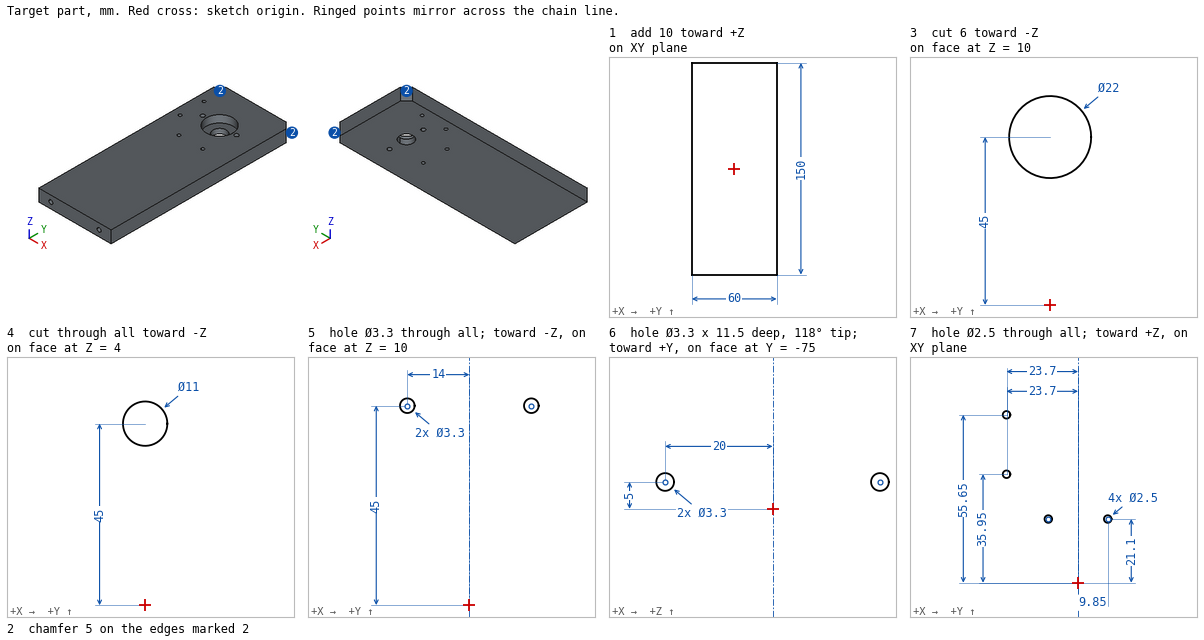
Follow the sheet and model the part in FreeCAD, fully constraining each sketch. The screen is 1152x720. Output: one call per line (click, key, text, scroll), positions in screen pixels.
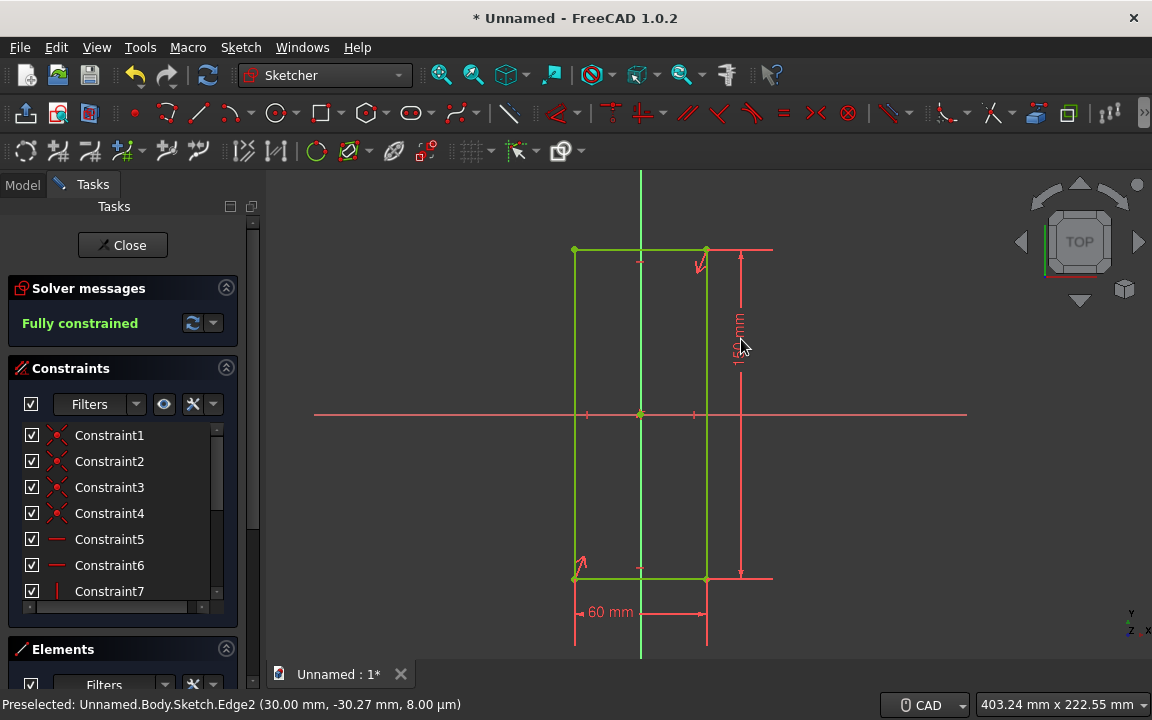
click(123, 245)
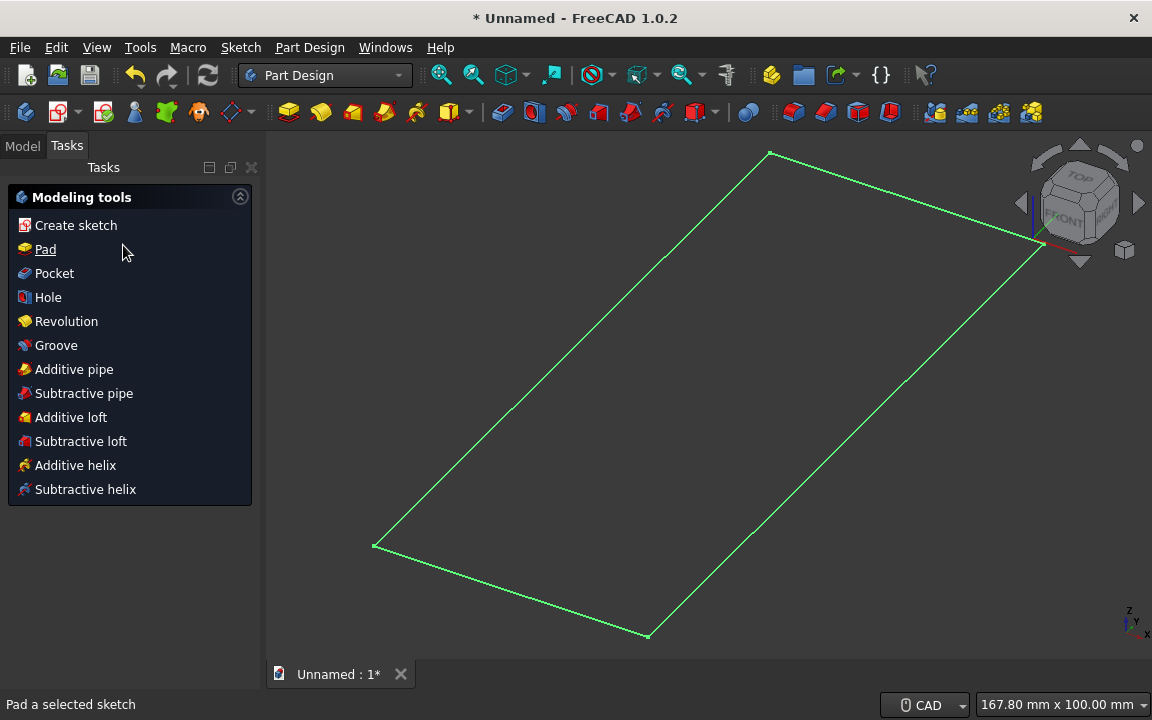
click(290, 112)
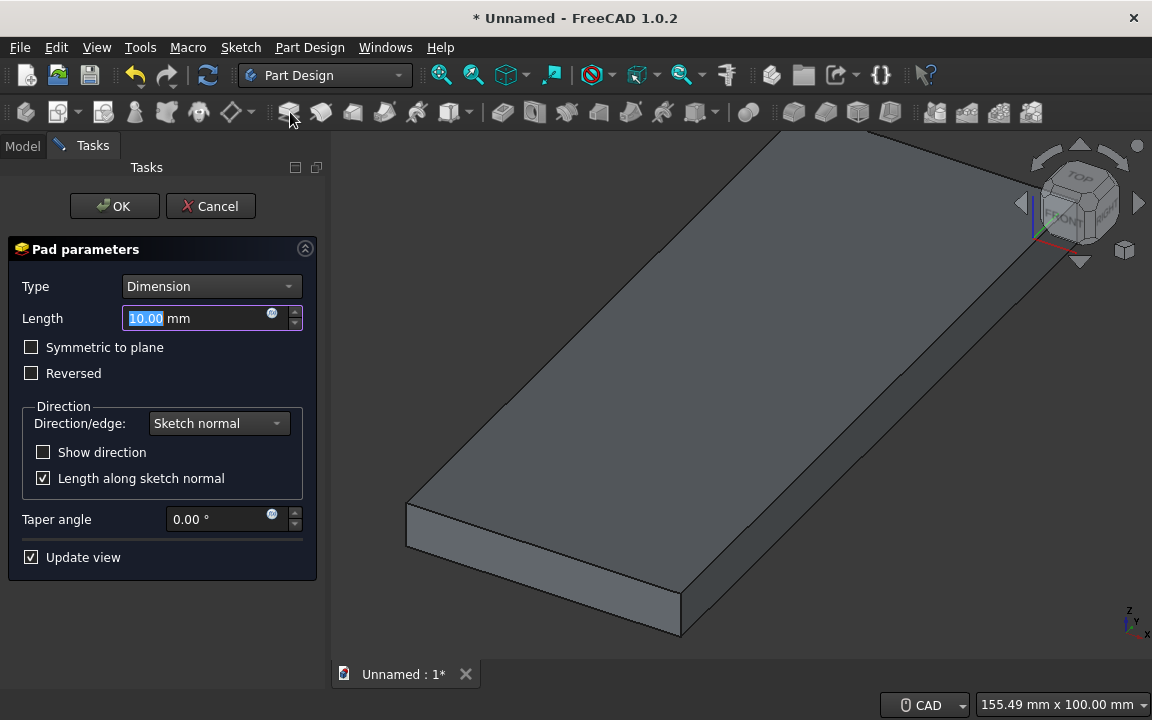
text(10)
key(Tab)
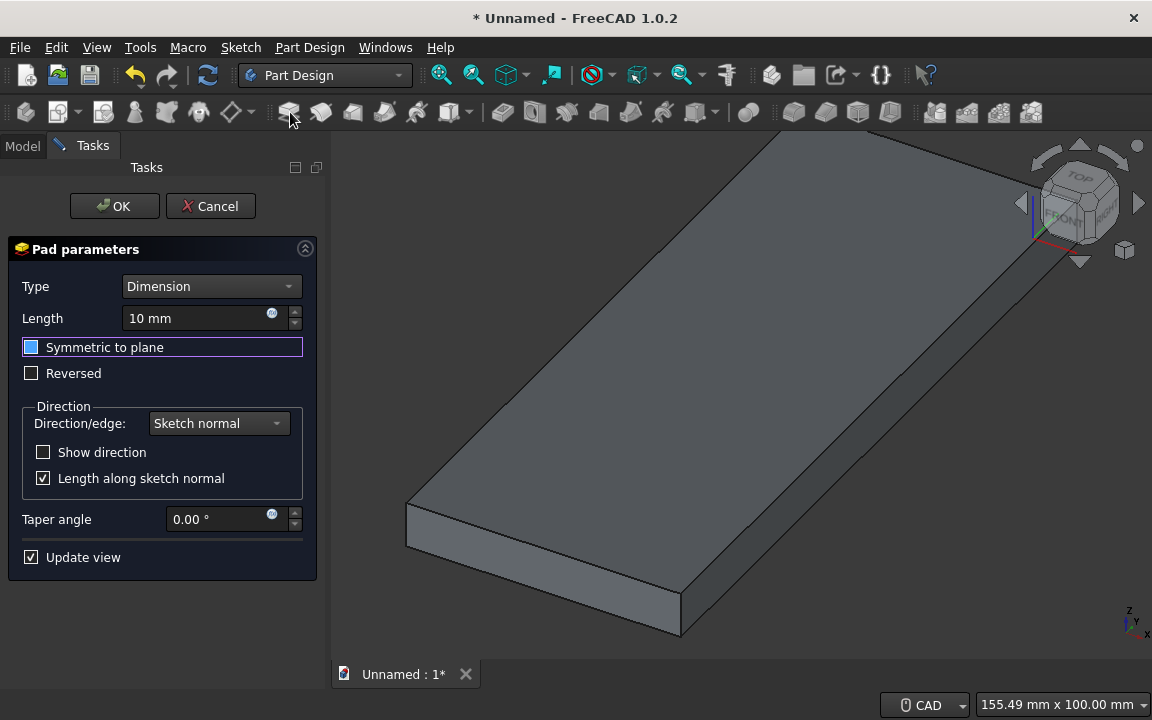
click(115, 206)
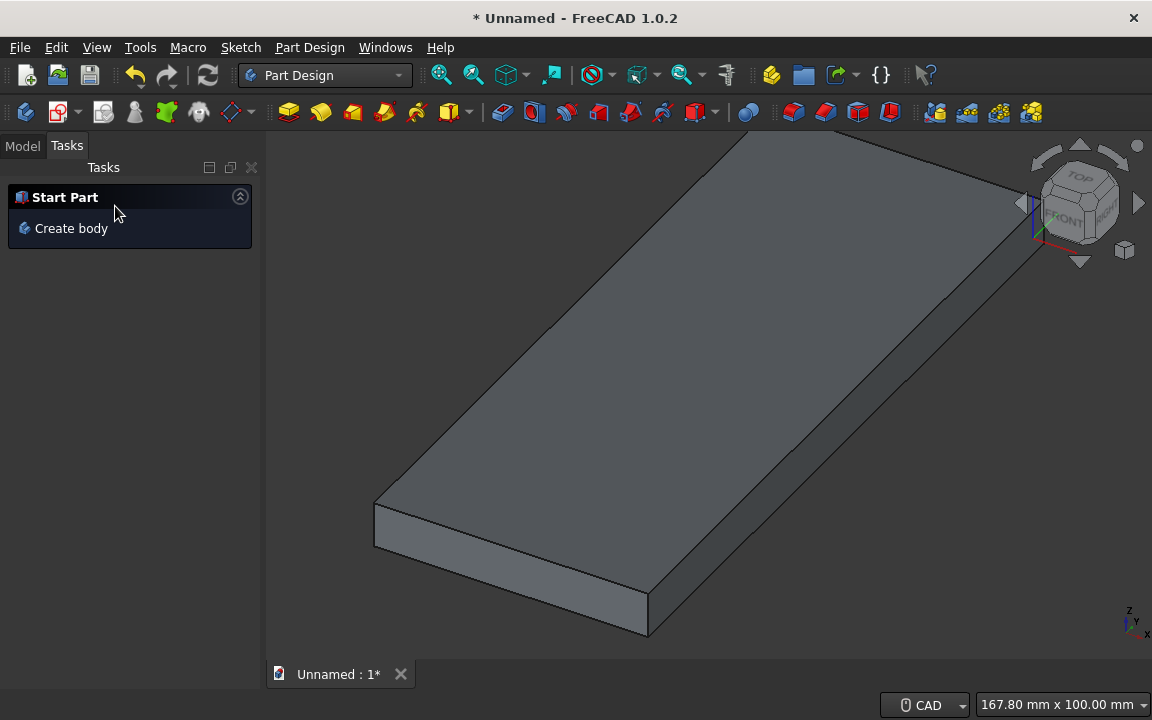
click(442, 76)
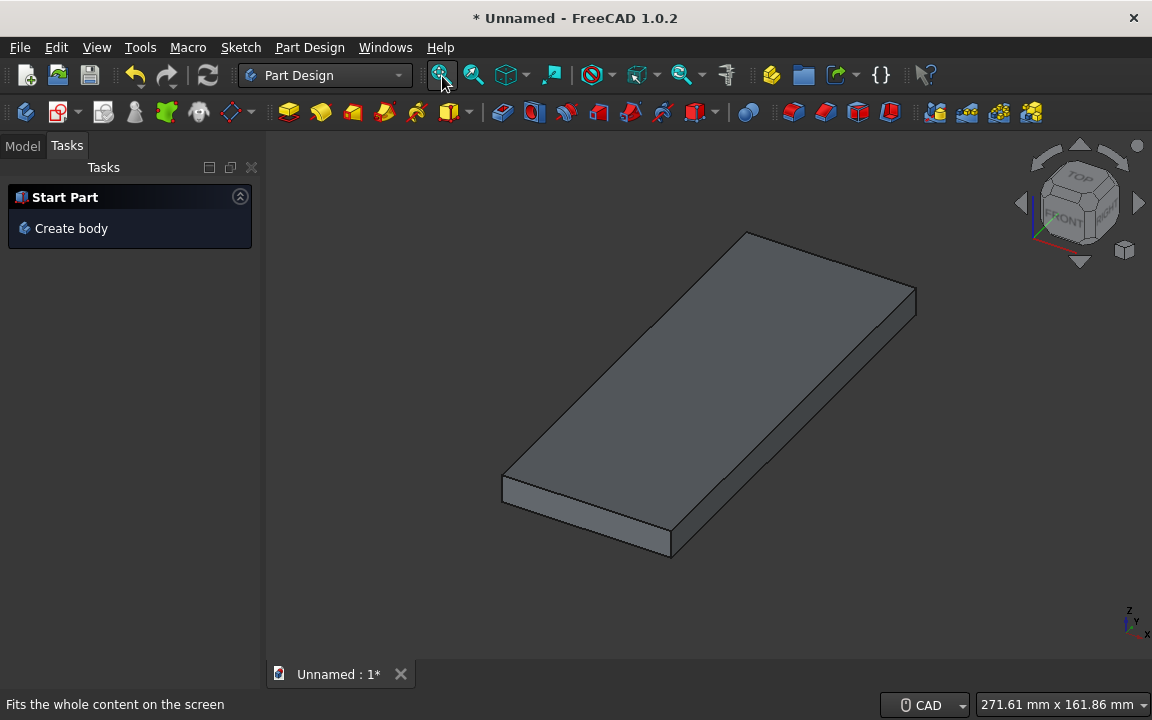
key(0)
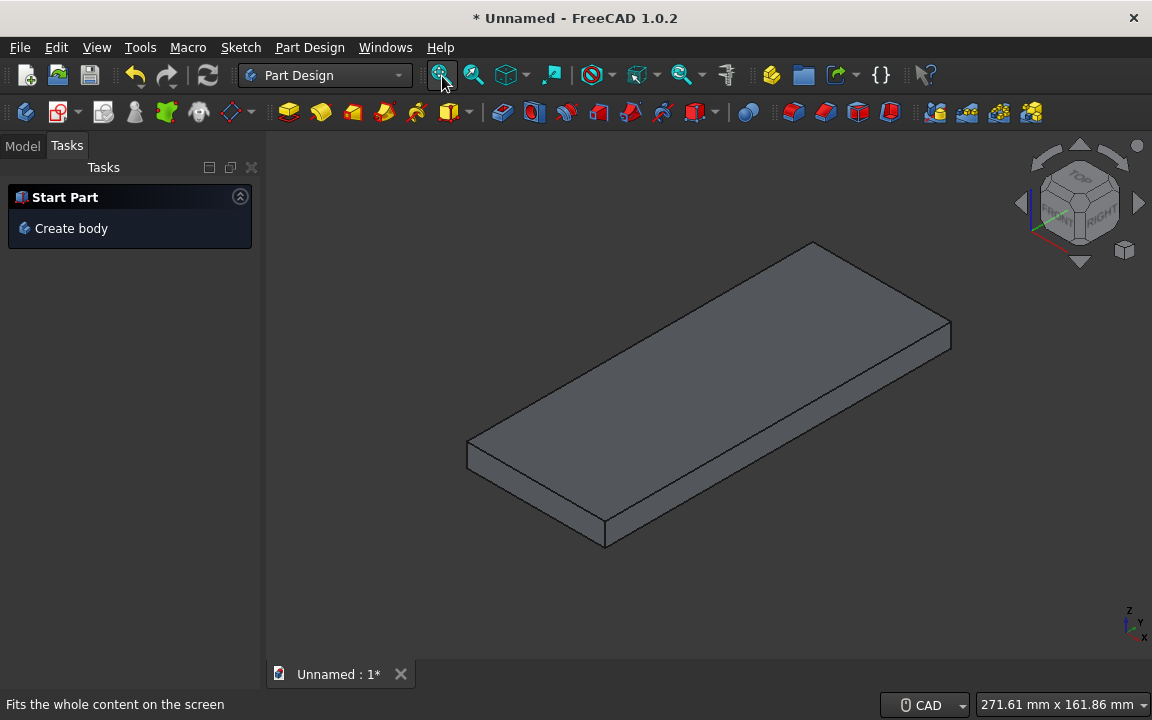
key(2)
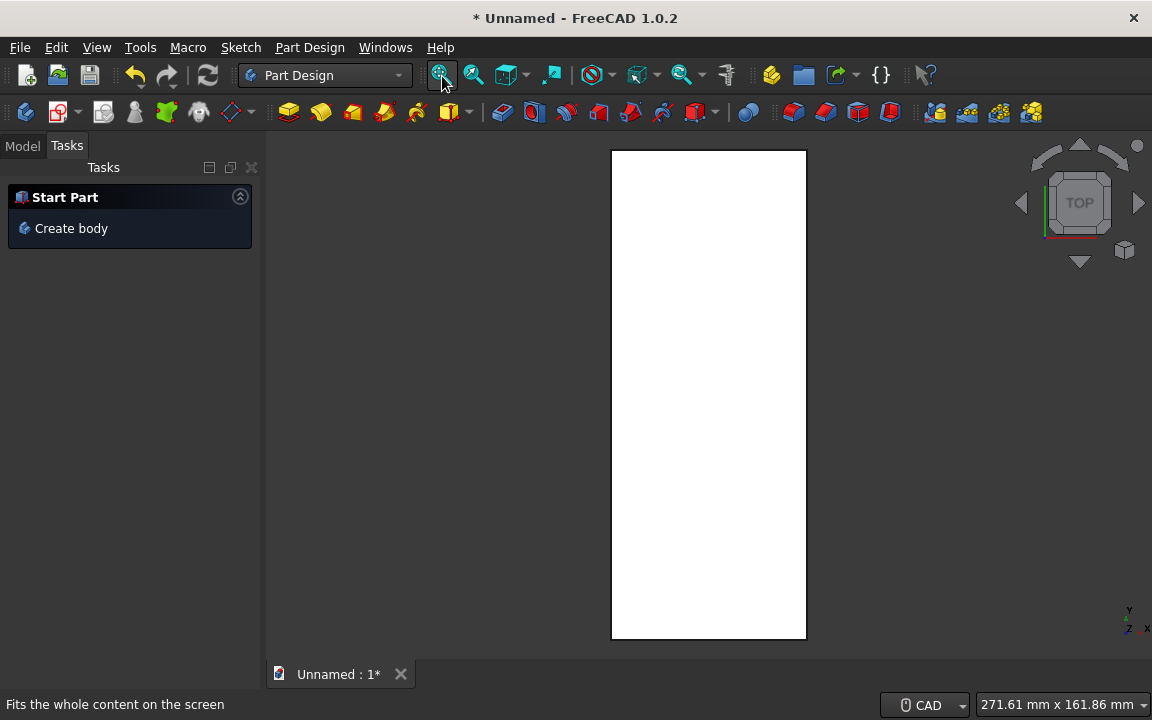
key(1)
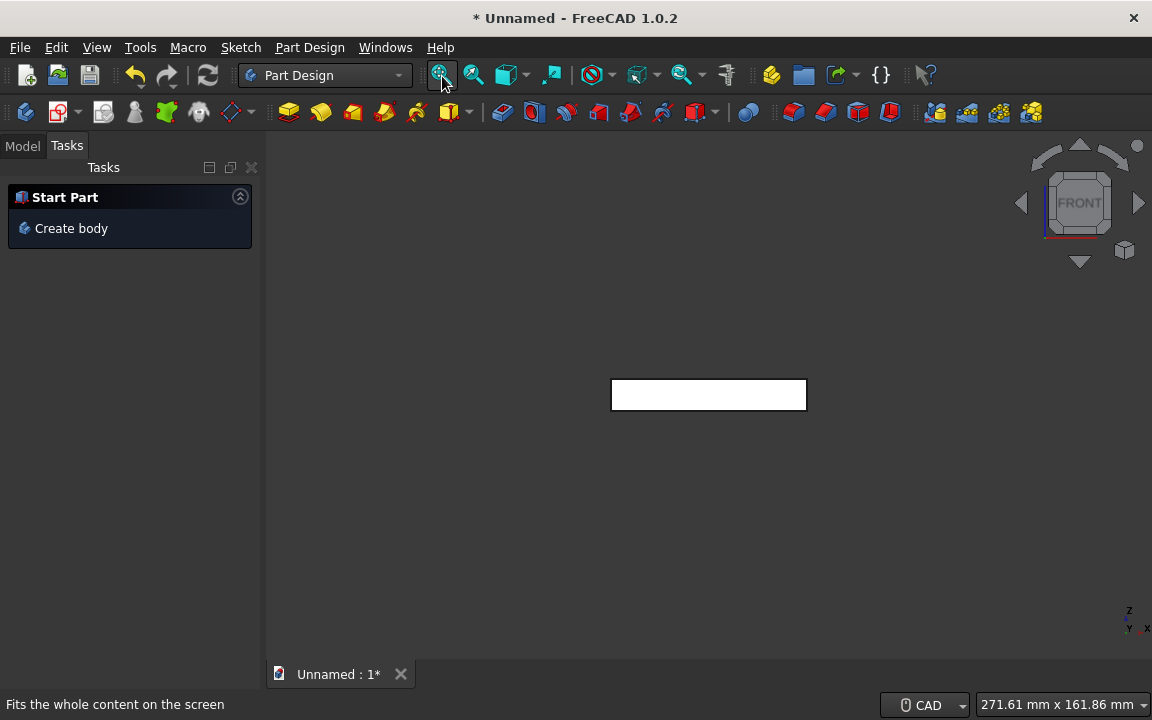
click(442, 76)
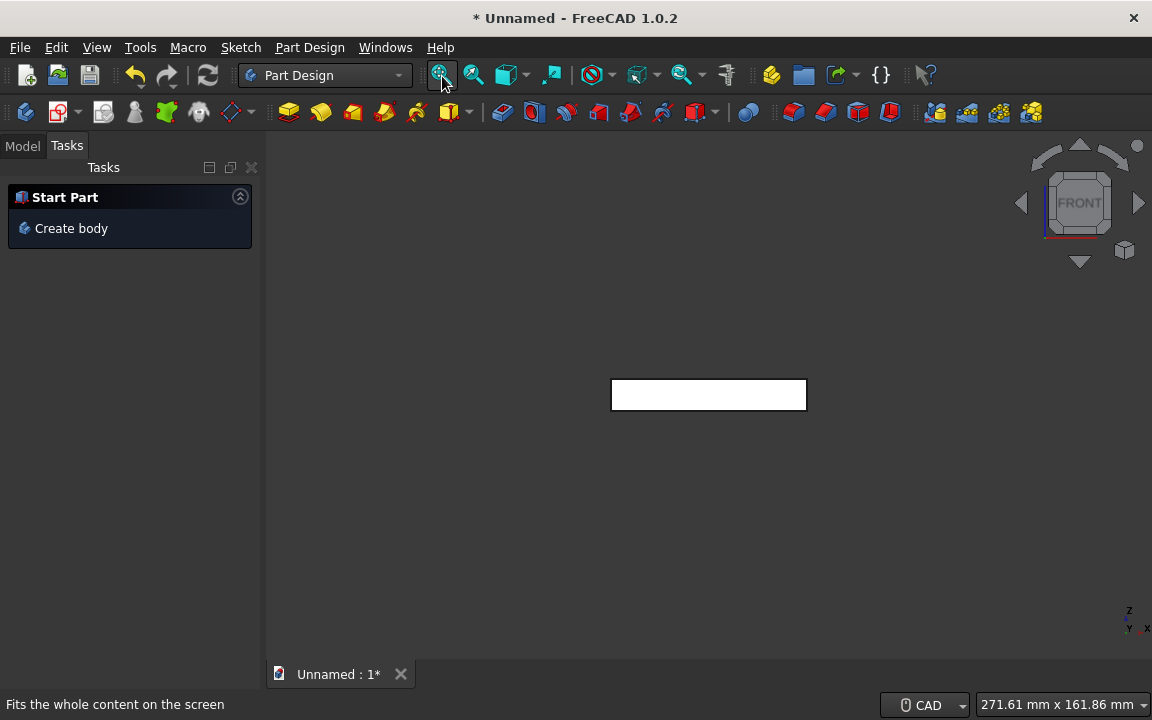
key(3)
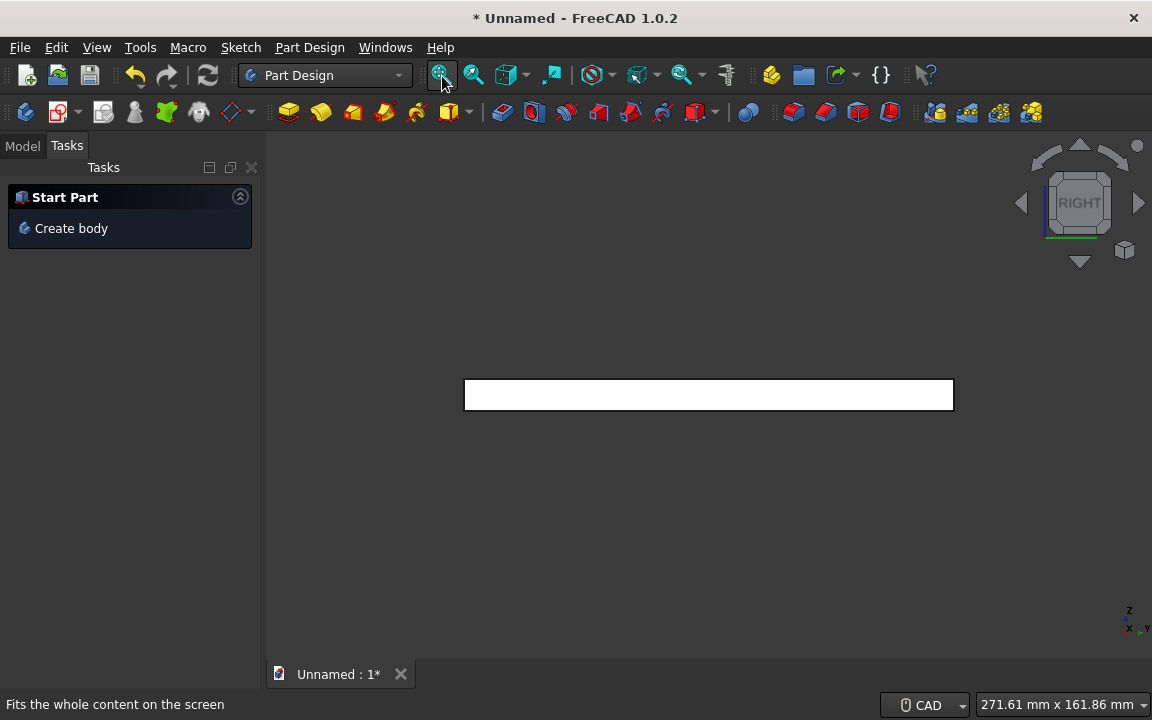
click(954, 394)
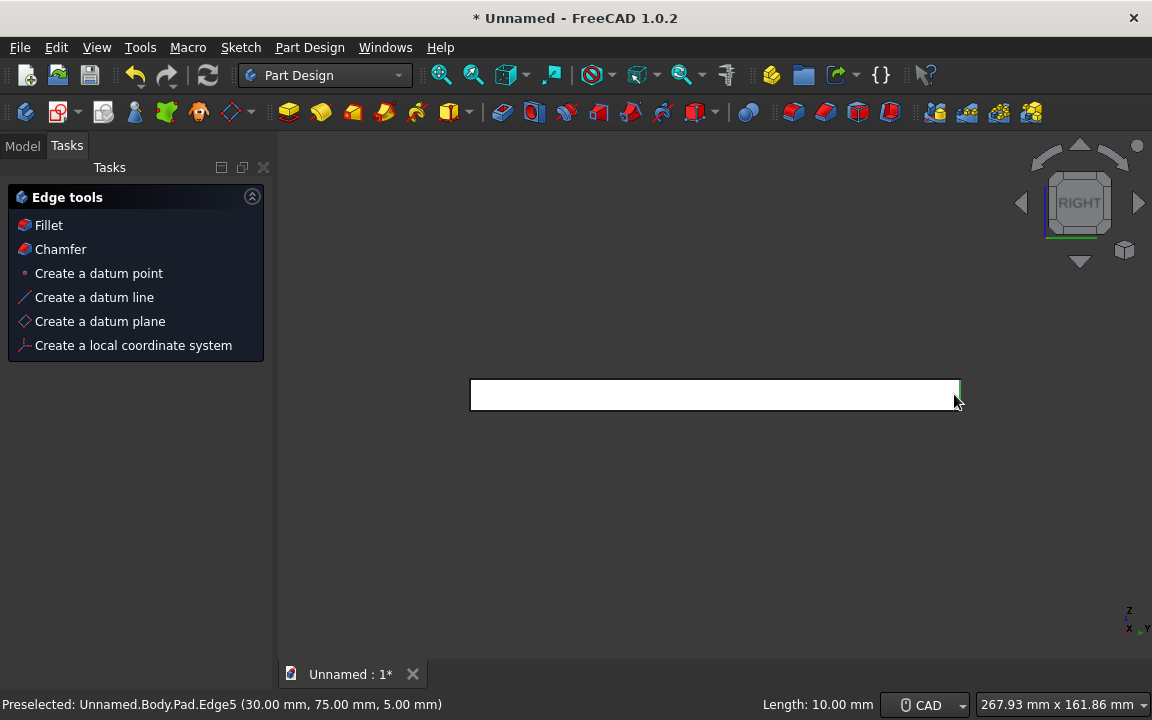
key(5)